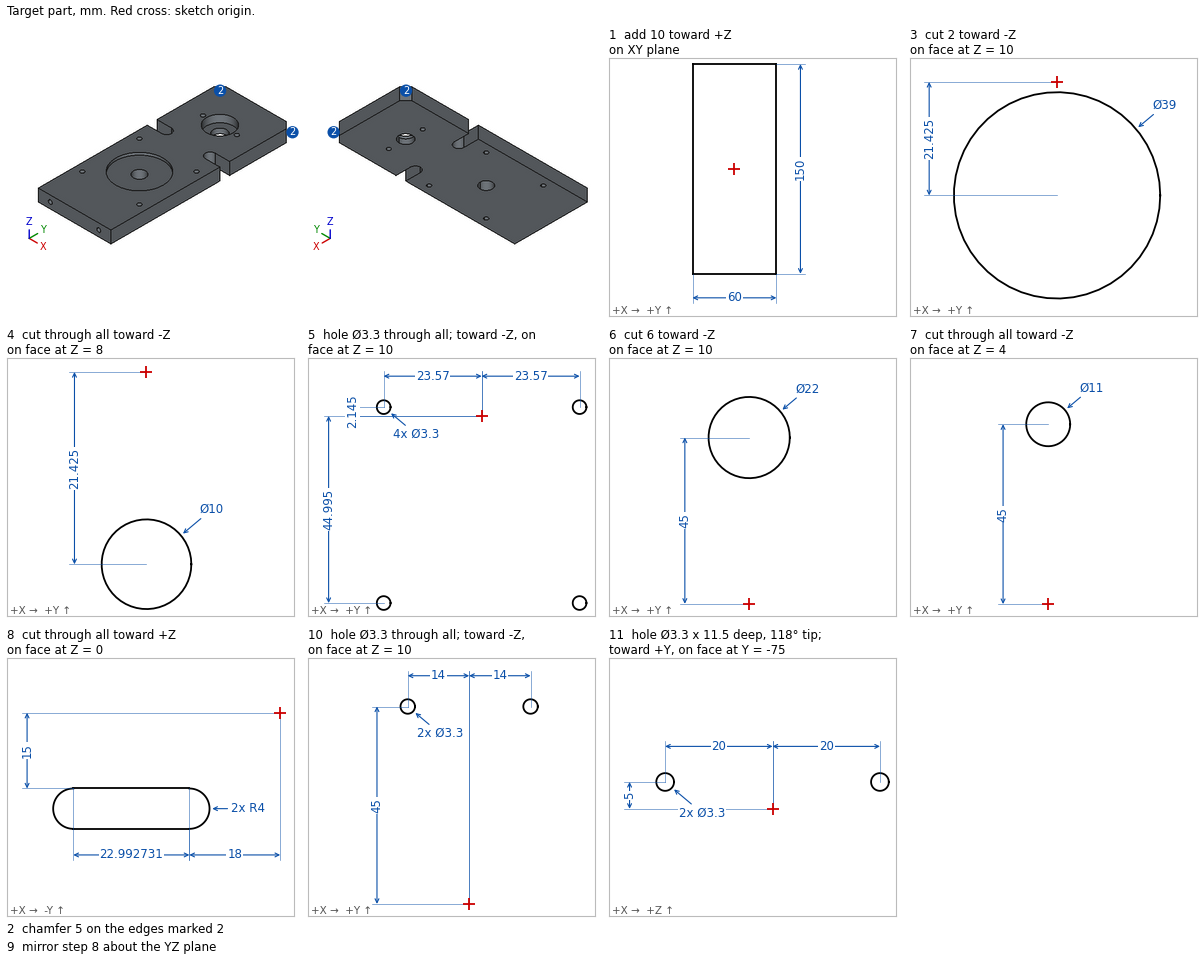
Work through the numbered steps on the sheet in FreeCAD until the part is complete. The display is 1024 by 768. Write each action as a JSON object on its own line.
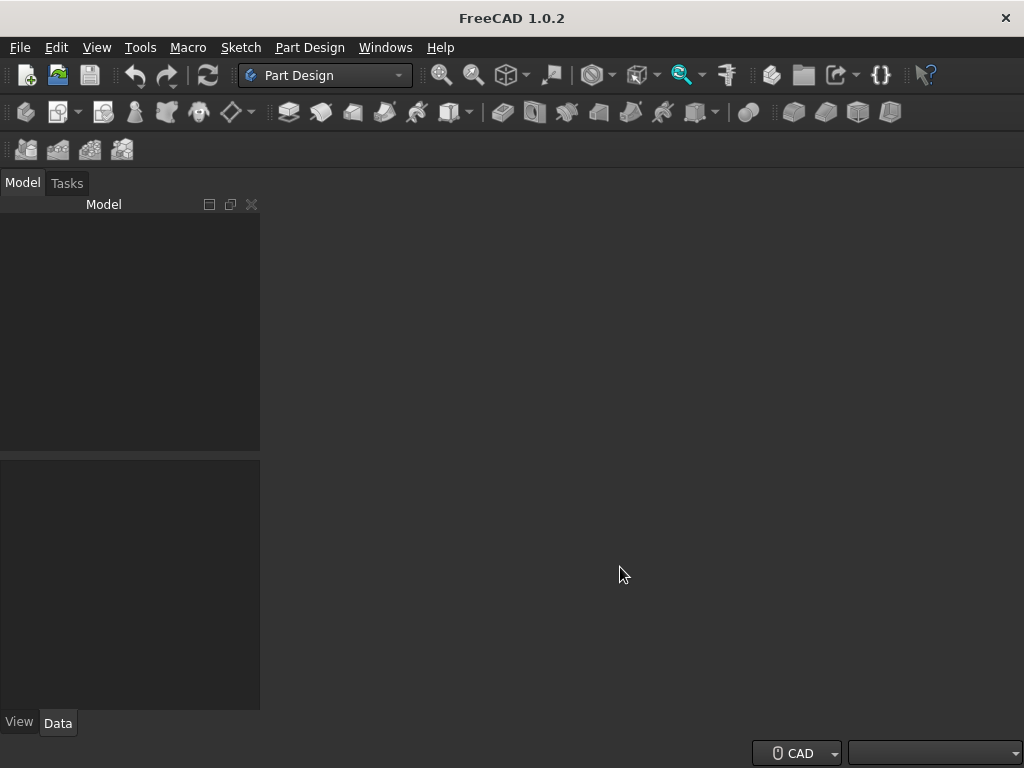
{"action": "left_click", "coordinate": [26, 76]}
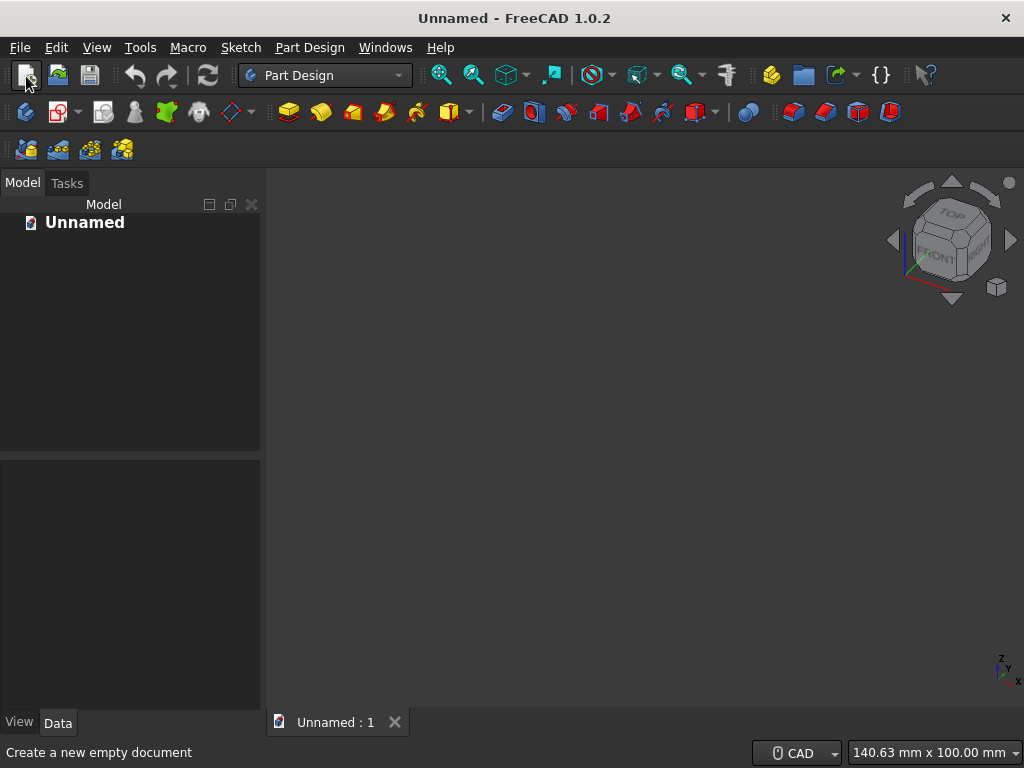
{"action": "left_click", "coordinate": [58, 112]}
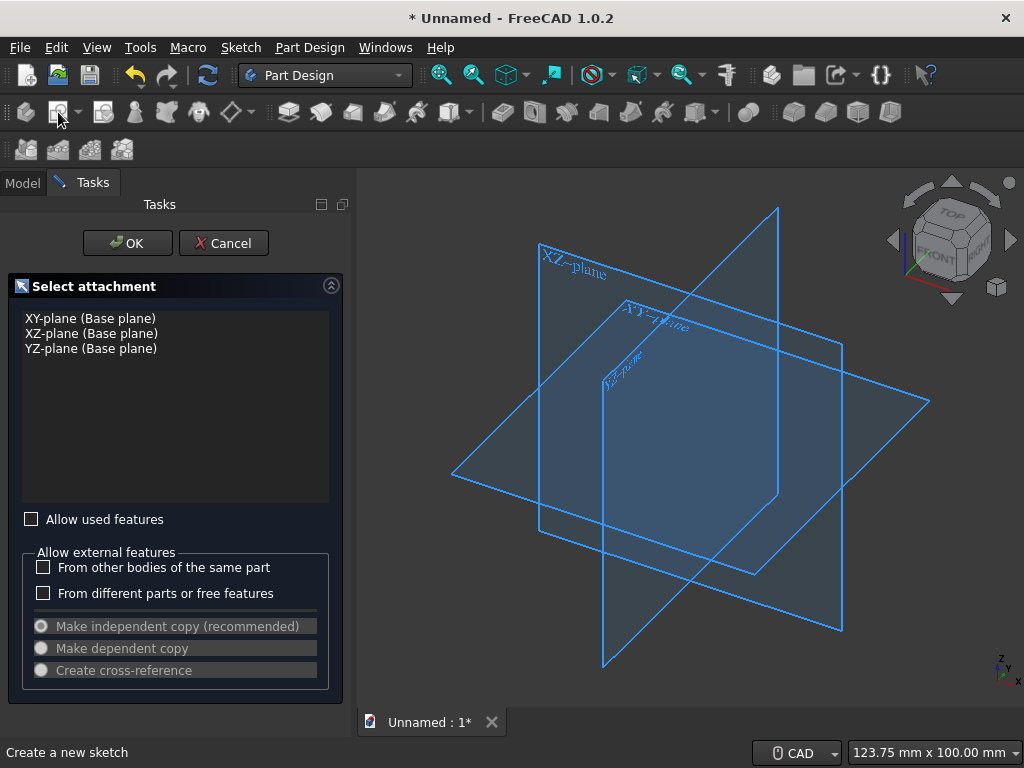
{"action": "left_click", "coordinate": [82, 318]}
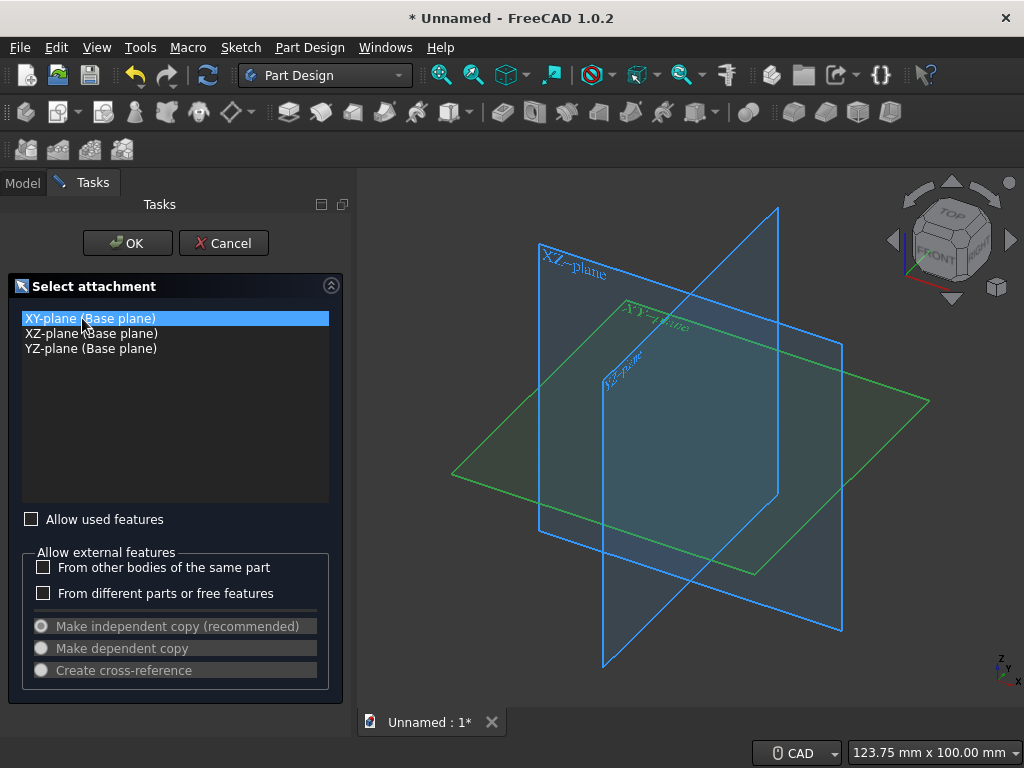
{"action": "left_click", "coordinate": [128, 243]}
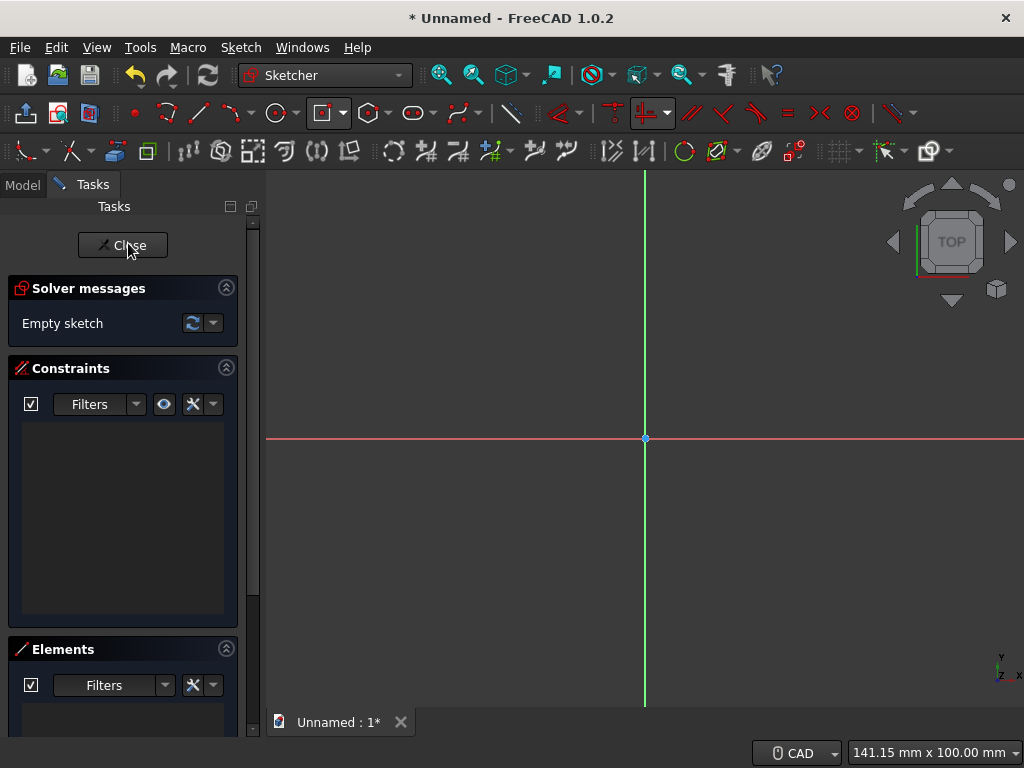
{"action": "scroll", "coordinate": [521, 438], "scroll_direction": "down", "scroll_amount": 4}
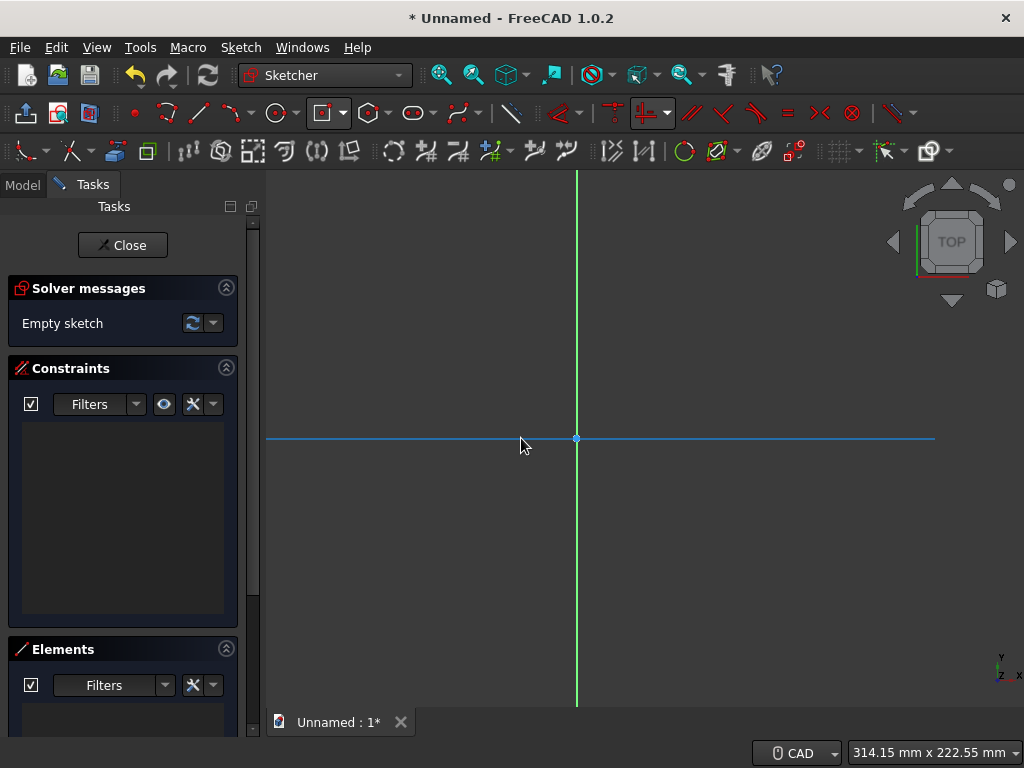
{"action": "left_click", "coordinate": [322, 114]}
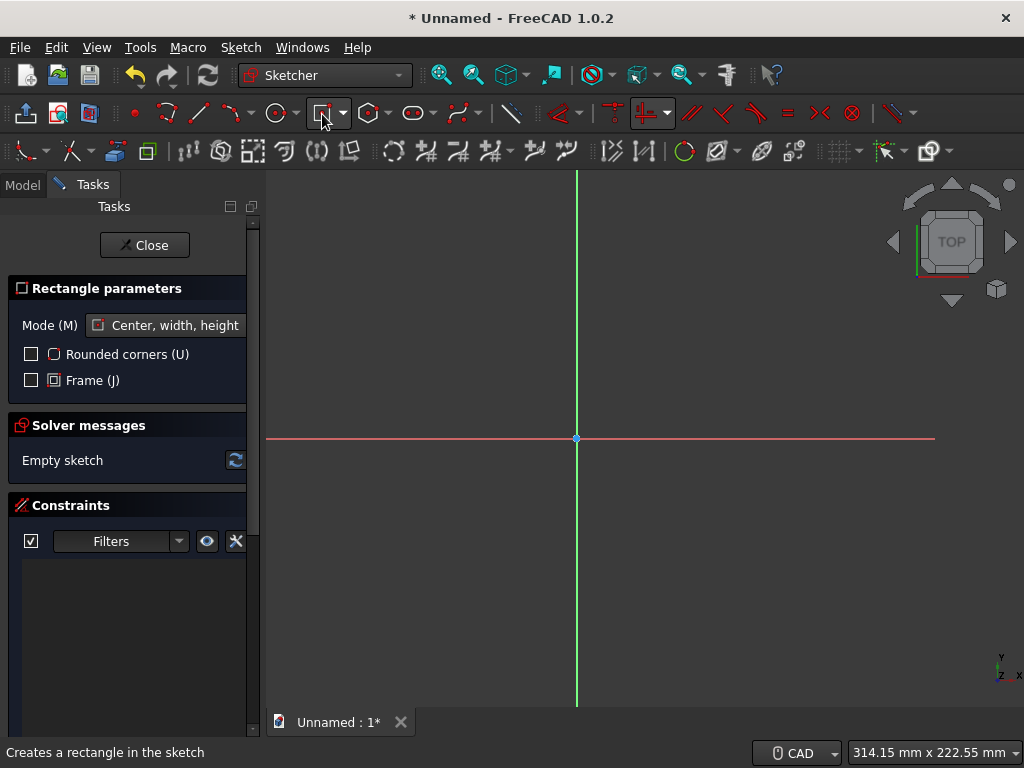
{"action": "left_click", "coordinate": [577, 438]}
{"action": "left_click", "coordinate": [649, 258]}
{"action": "key", "text": "Escape"}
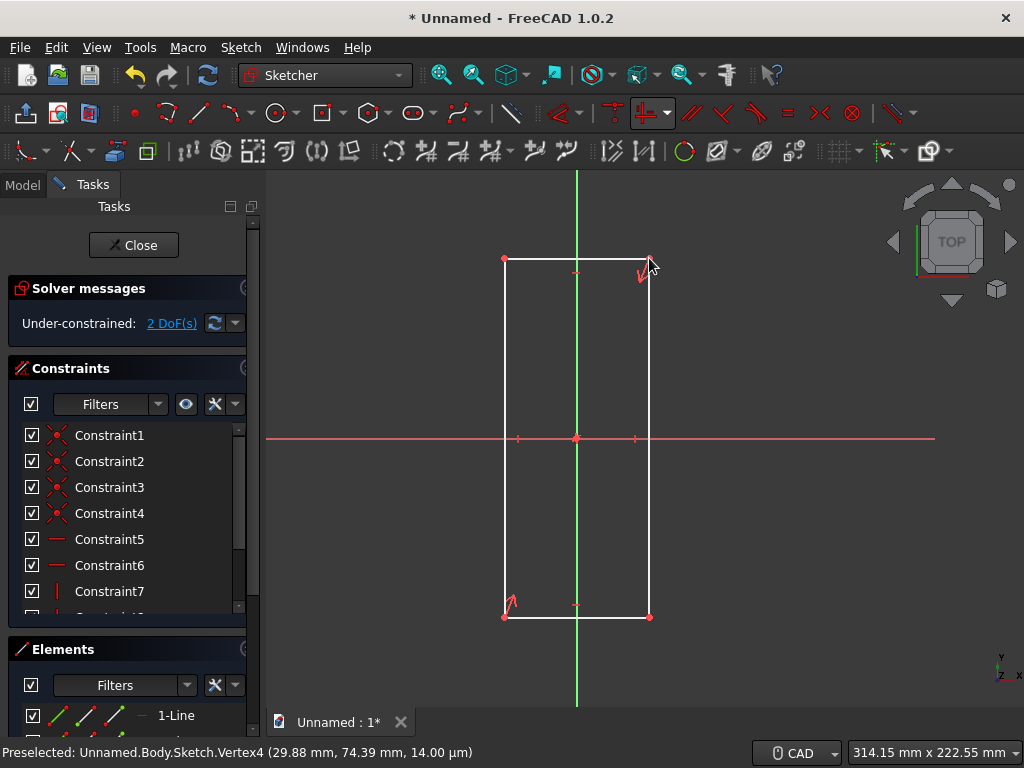
{"action": "left_click", "coordinate": [558, 114]}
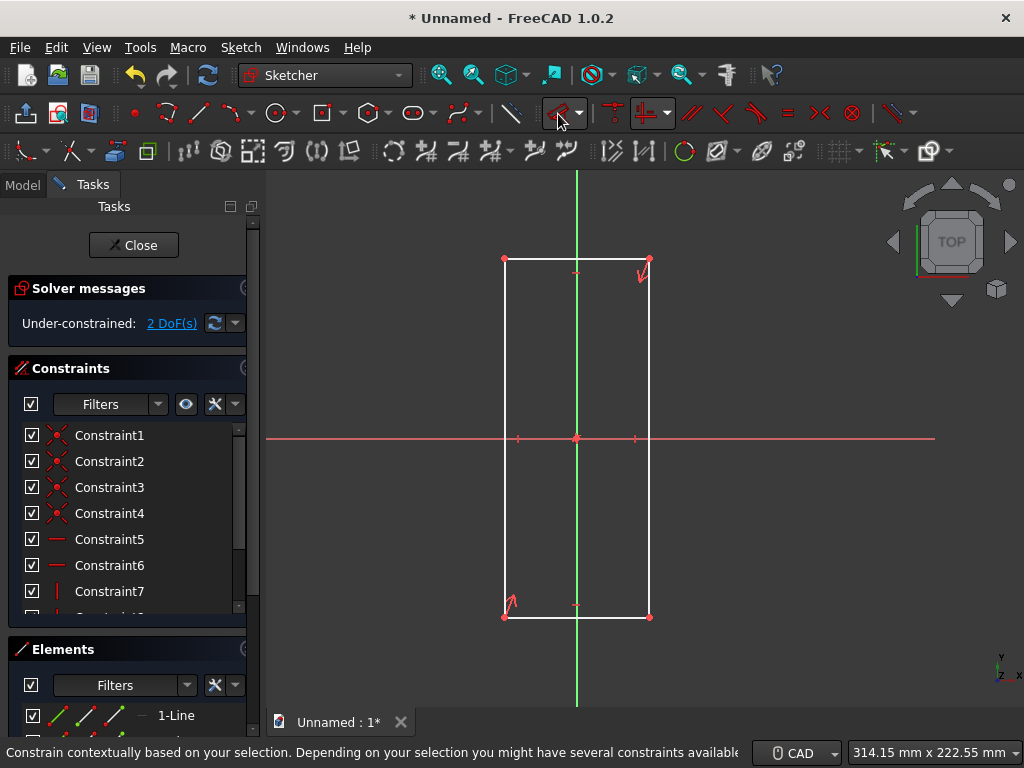
{"action": "left_click", "coordinate": [548, 618]}
{"action": "left_click", "coordinate": [544, 652]}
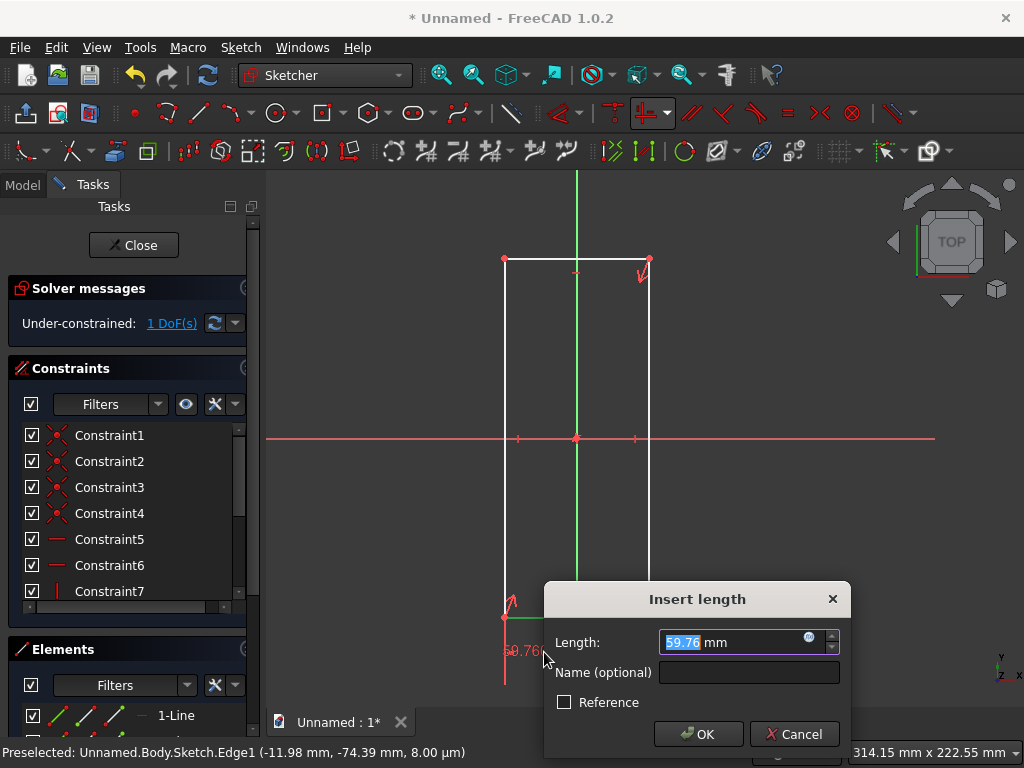
{"action": "type", "text": "60"}
{"action": "key", "text": "Return"}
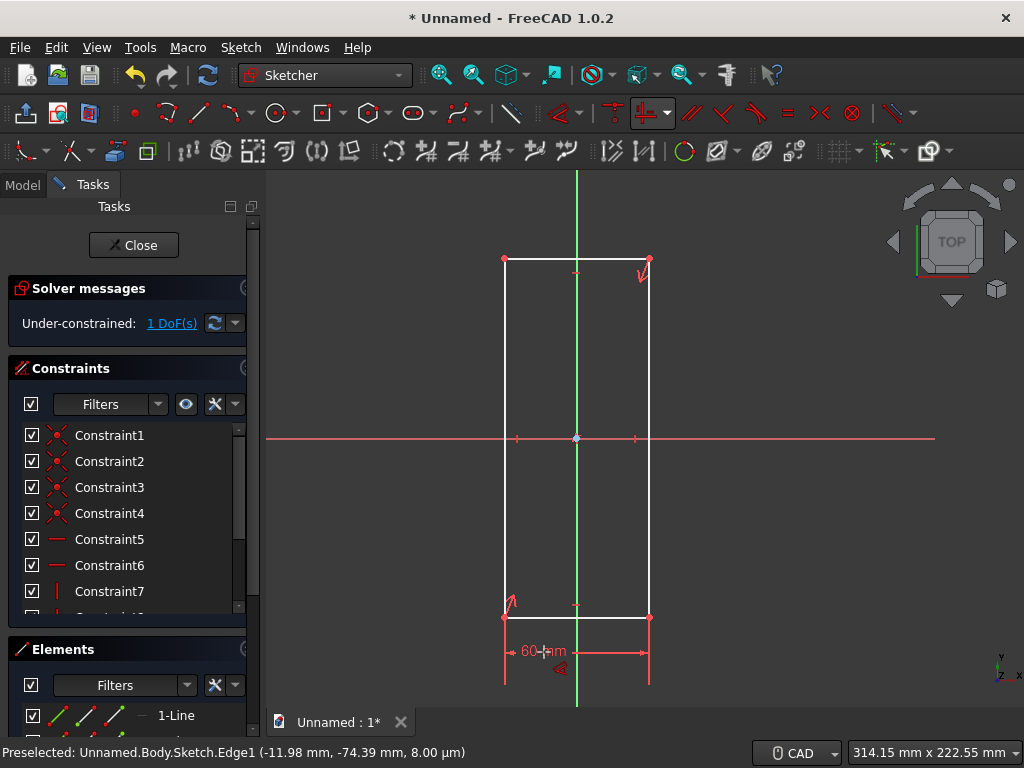
{"action": "left_click", "coordinate": [649, 510]}
{"action": "left_click", "coordinate": [683, 356]}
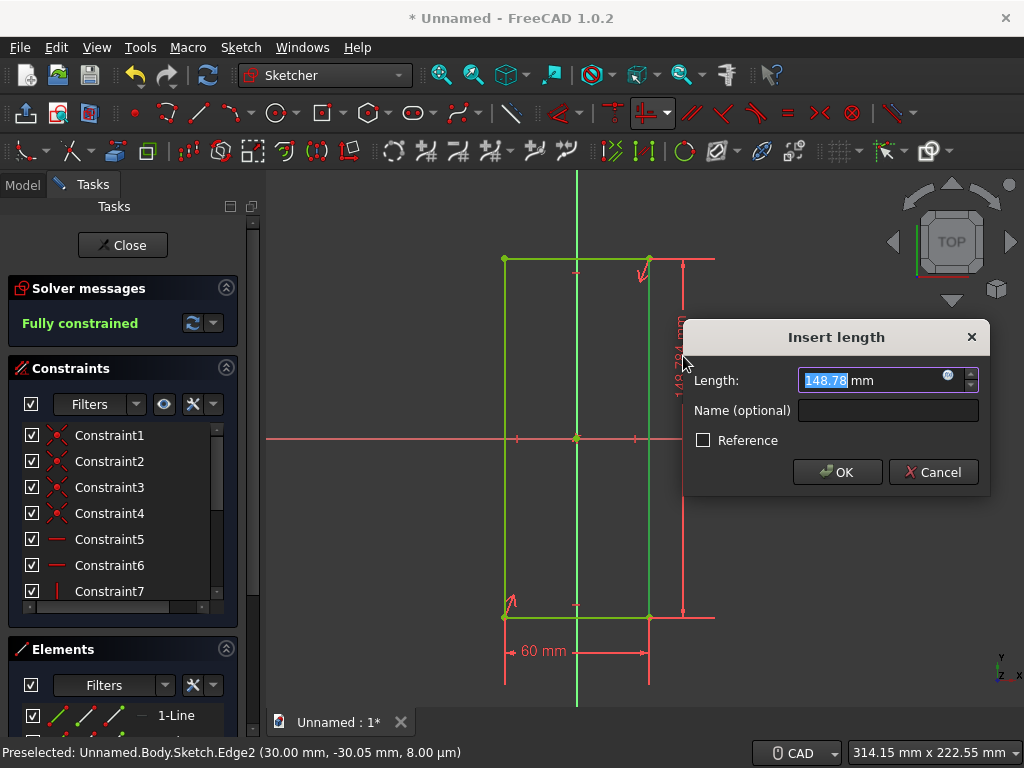
{"action": "type", "text": "150"}
{"action": "key", "text": "Return"}
{"action": "key", "text": "Escape"}